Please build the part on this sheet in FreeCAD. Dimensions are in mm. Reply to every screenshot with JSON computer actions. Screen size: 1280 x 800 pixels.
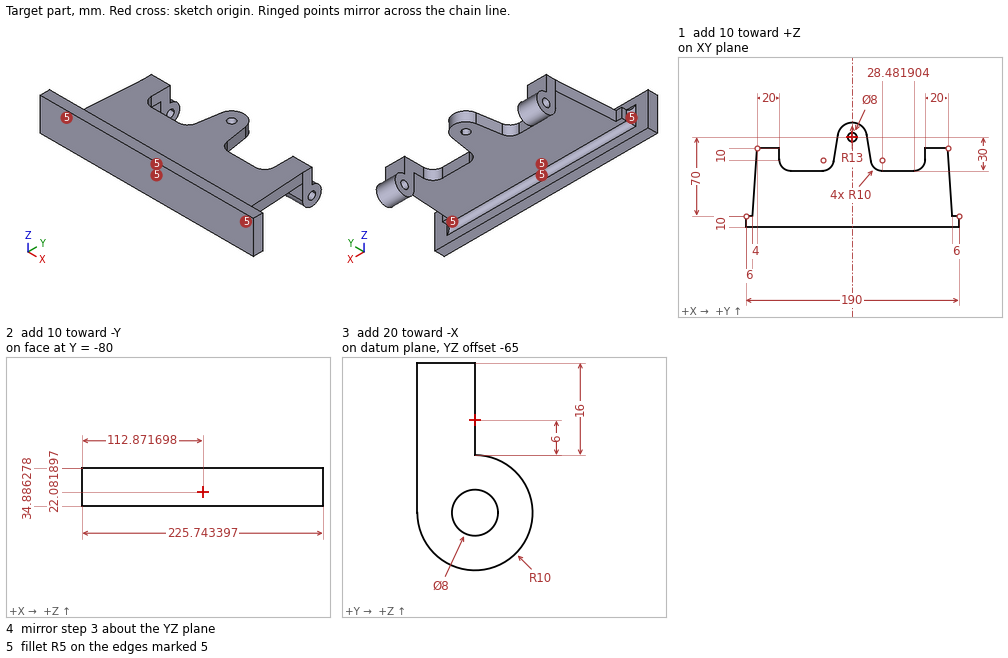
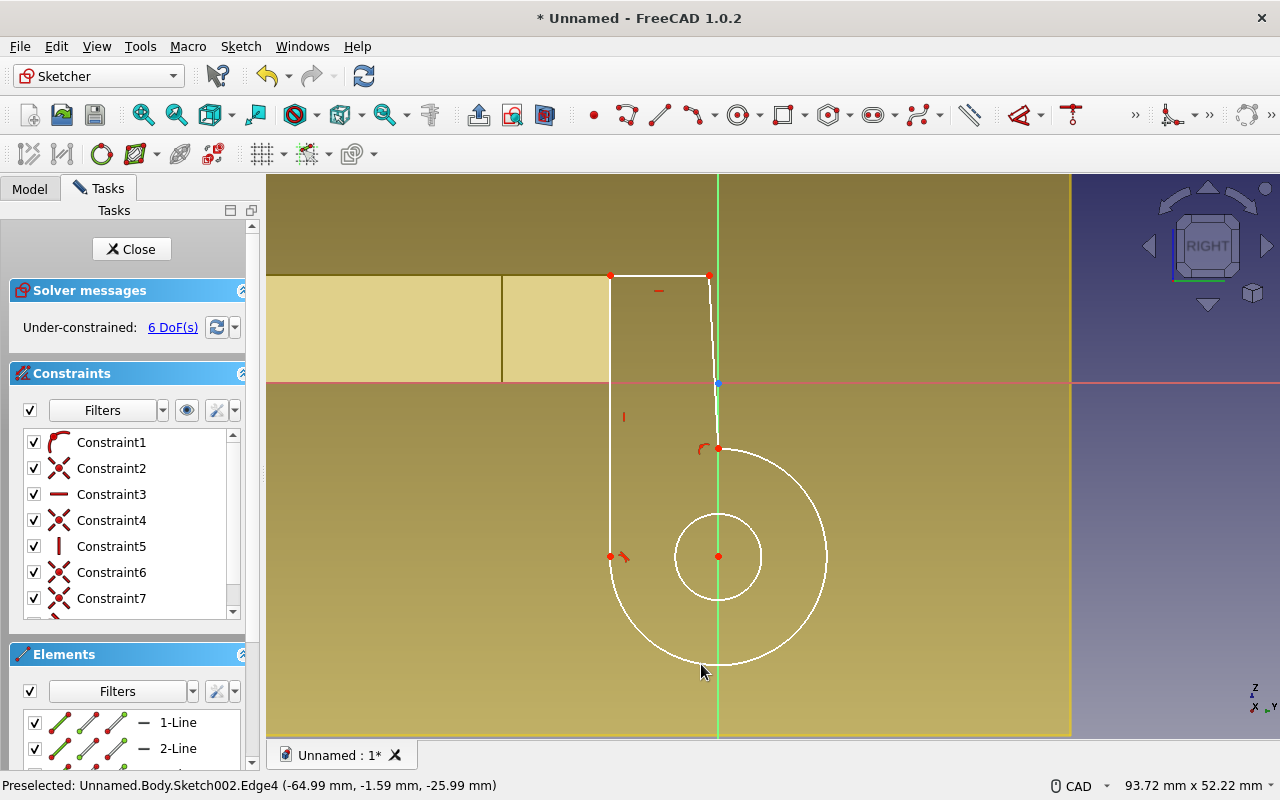
{"action": "left_click", "coordinate": [716, 397]}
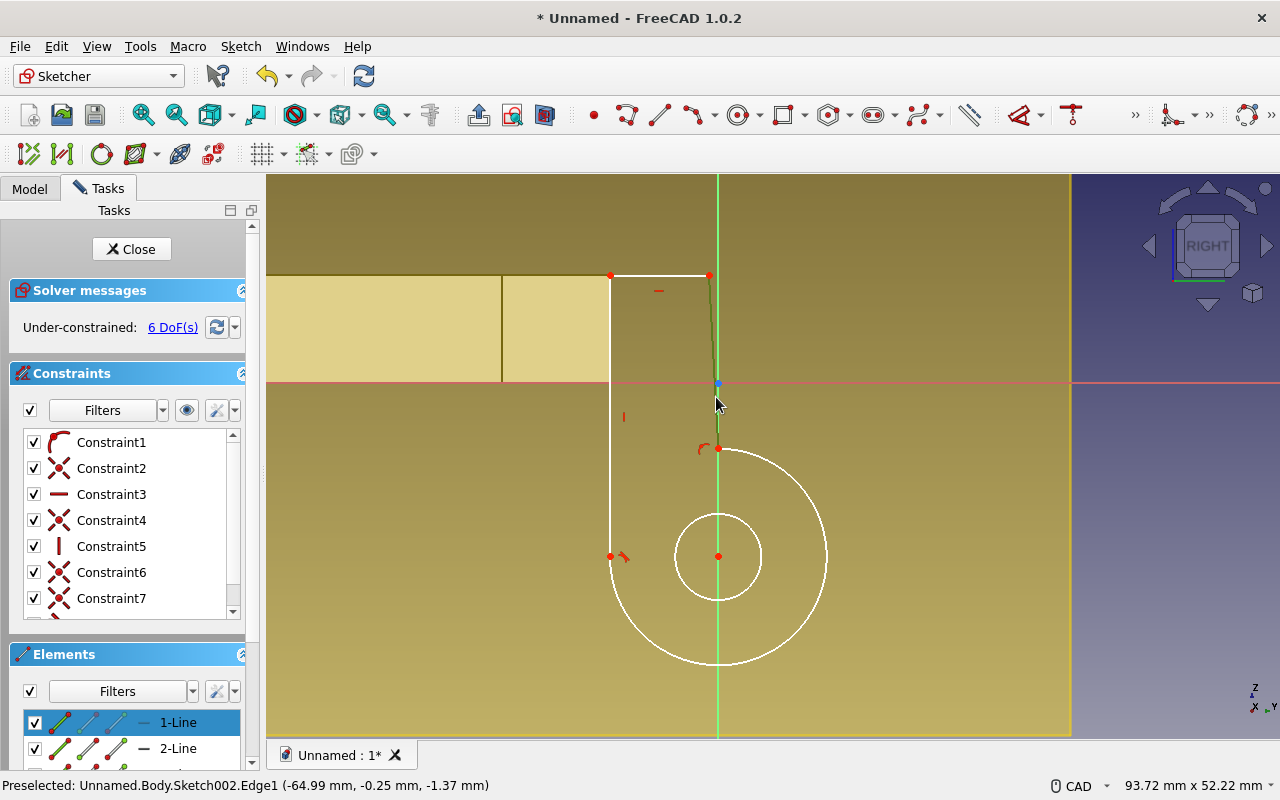
{"action": "key", "text": "v"}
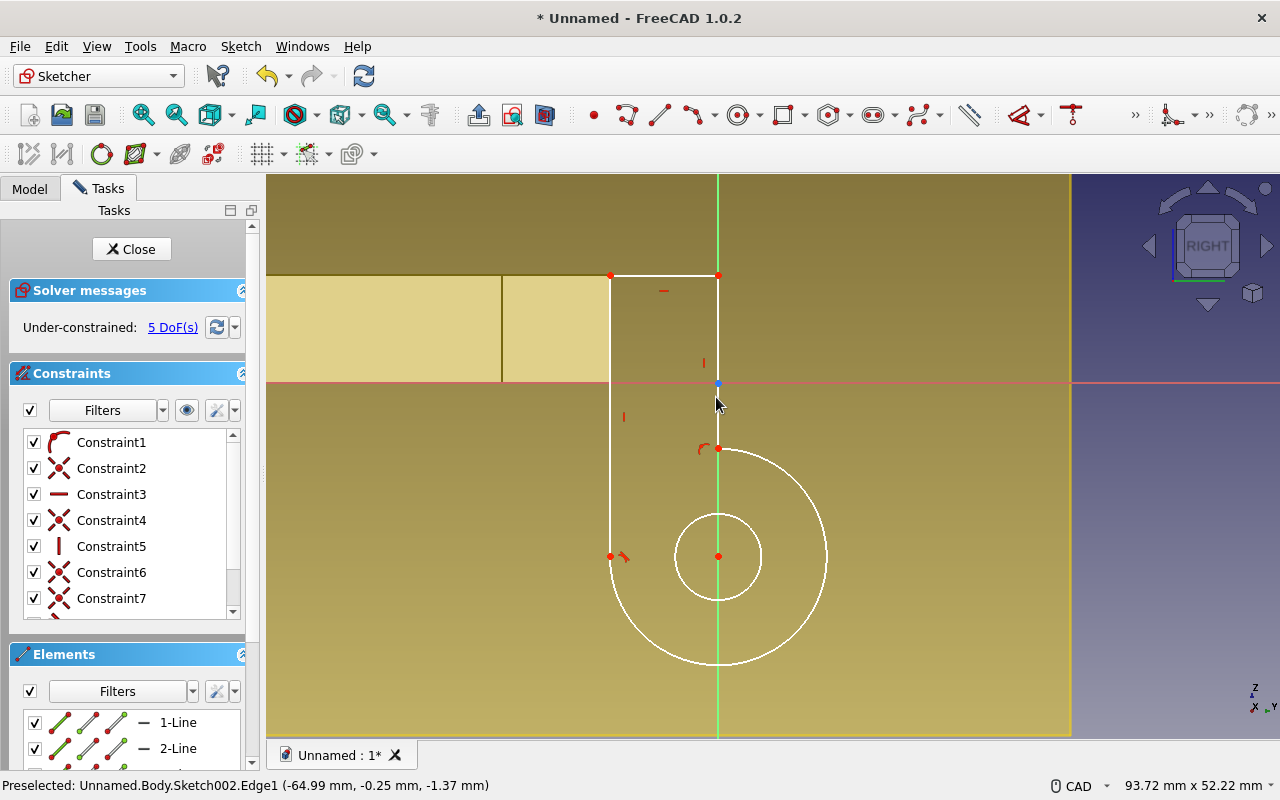
{"action": "left_click", "coordinate": [718, 557]}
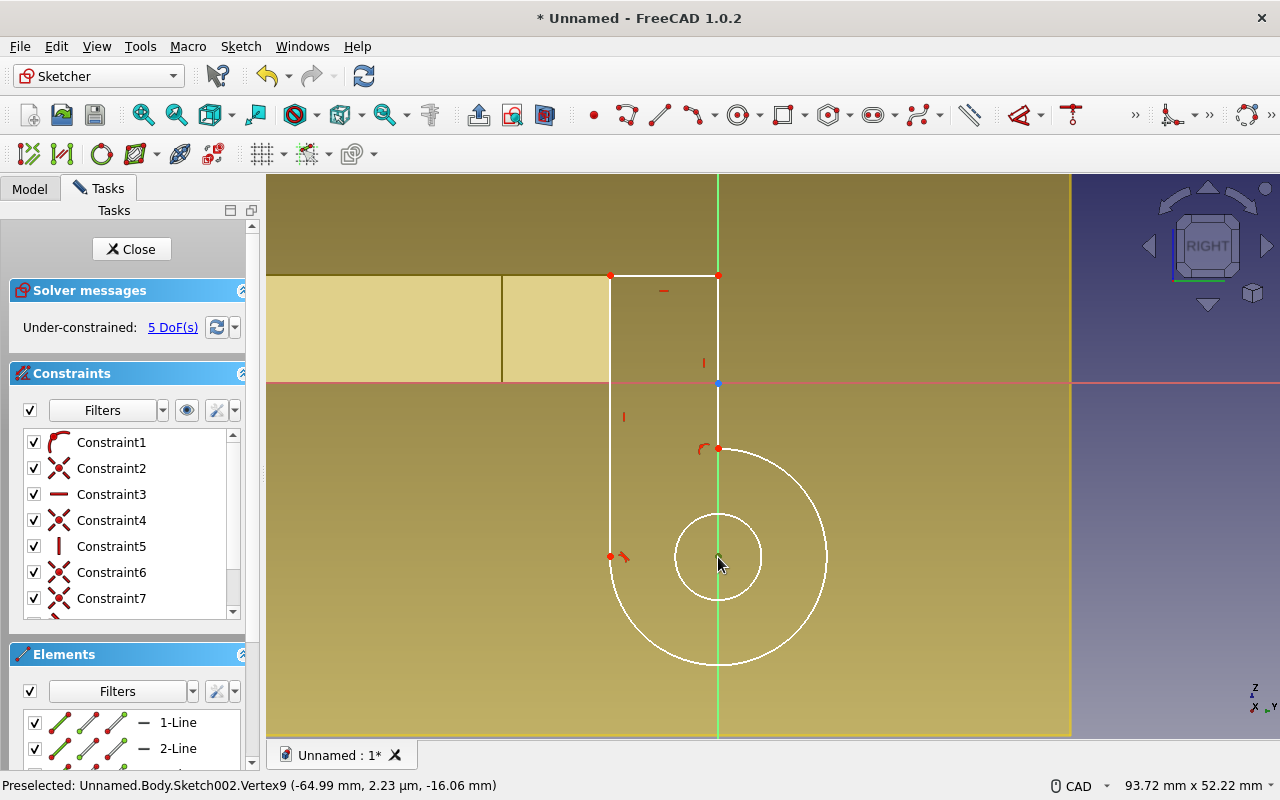
{"action": "left_click", "coordinate": [718, 566]}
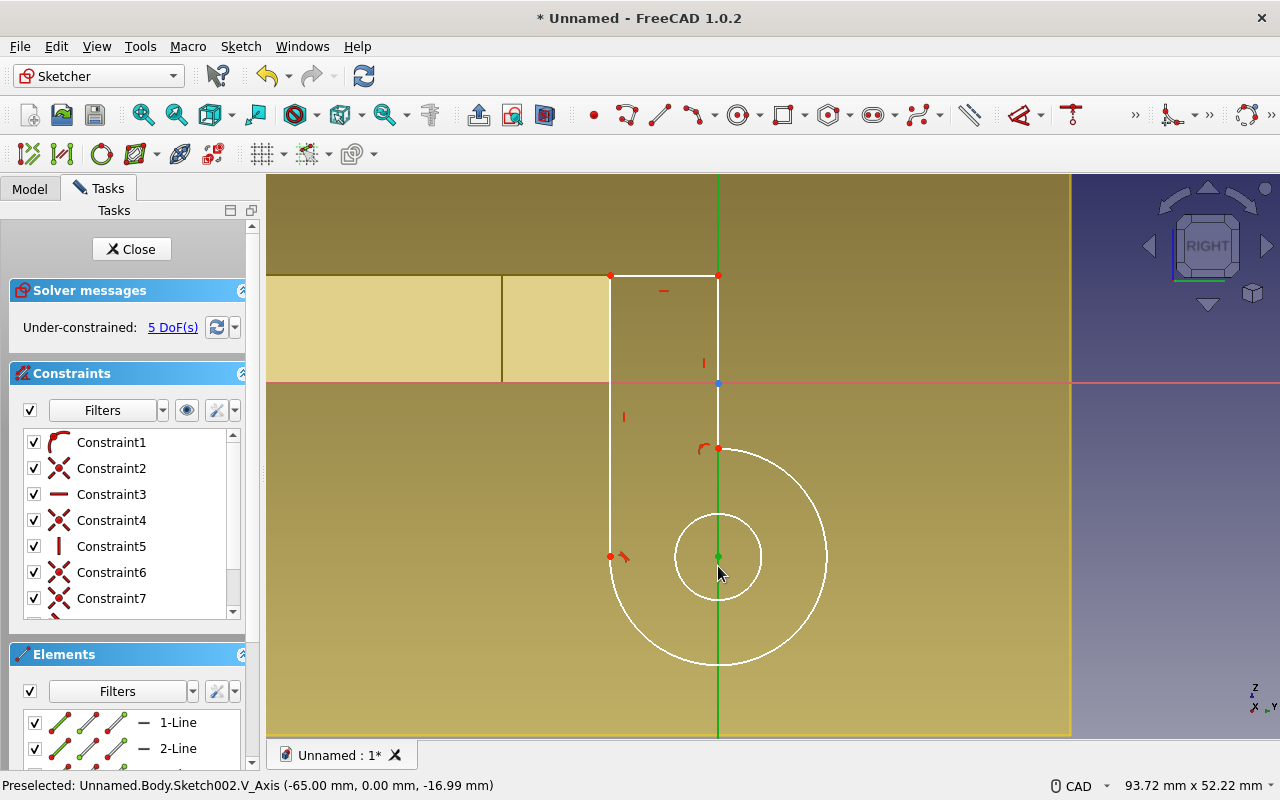
{"action": "left_click", "coordinate": [1071, 116]}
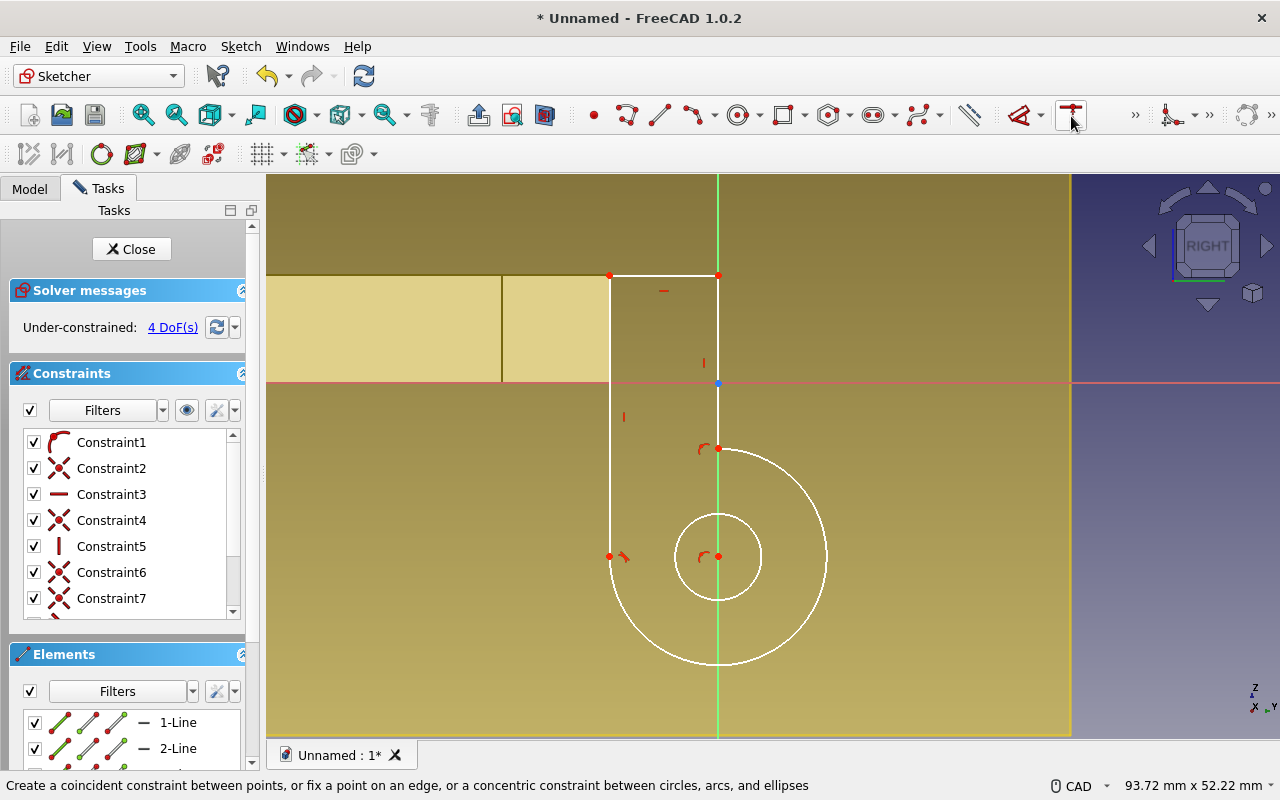
{"action": "key", "text": "d"}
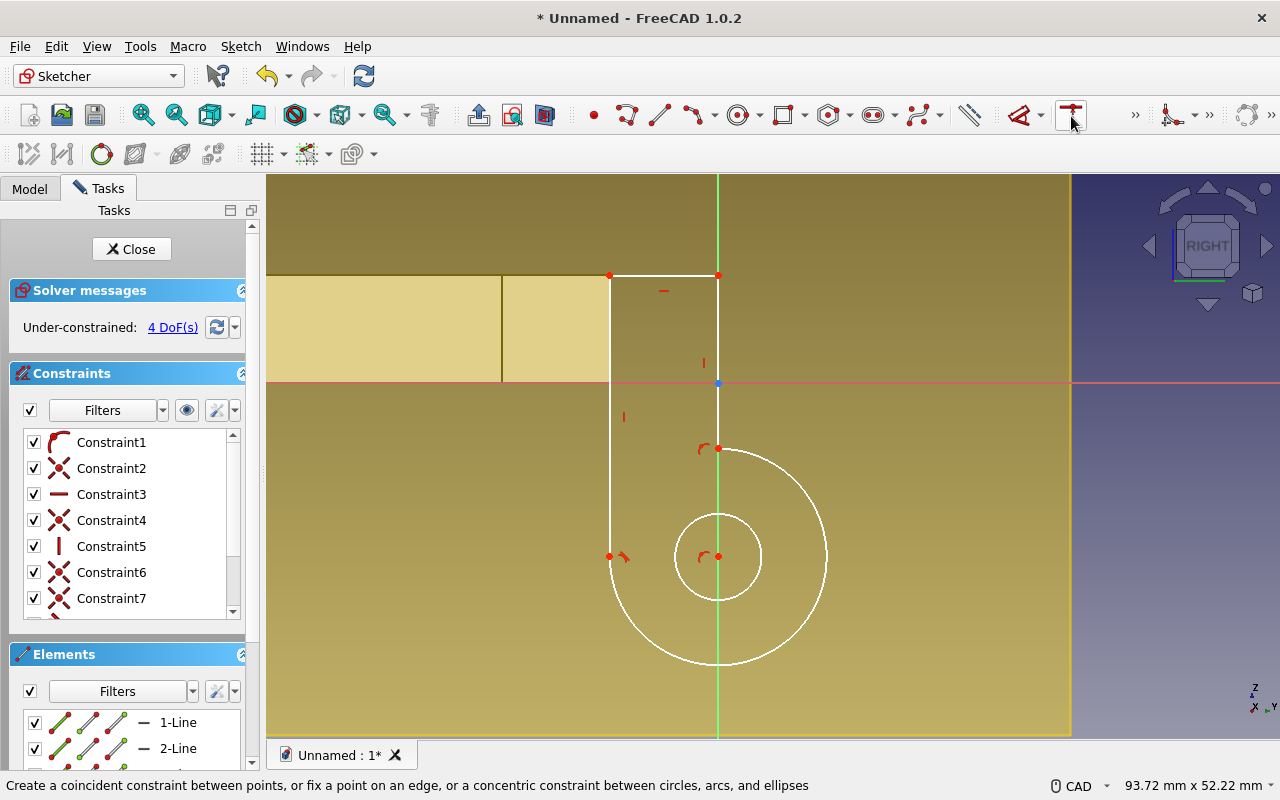
{"action": "left_click", "coordinate": [701, 664]}
{"action": "left_click", "coordinate": [696, 696]}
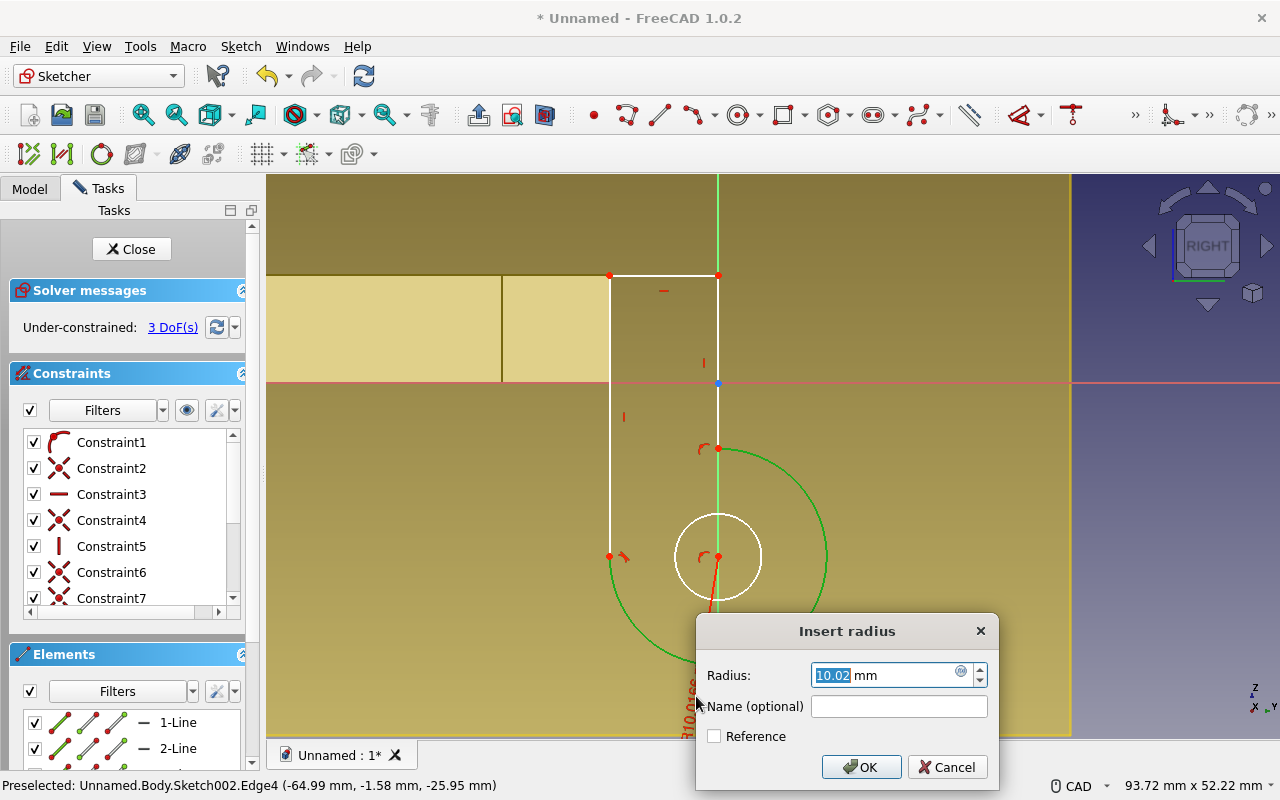
{"action": "type", "text": "10"}
{"action": "key", "text": "Return"}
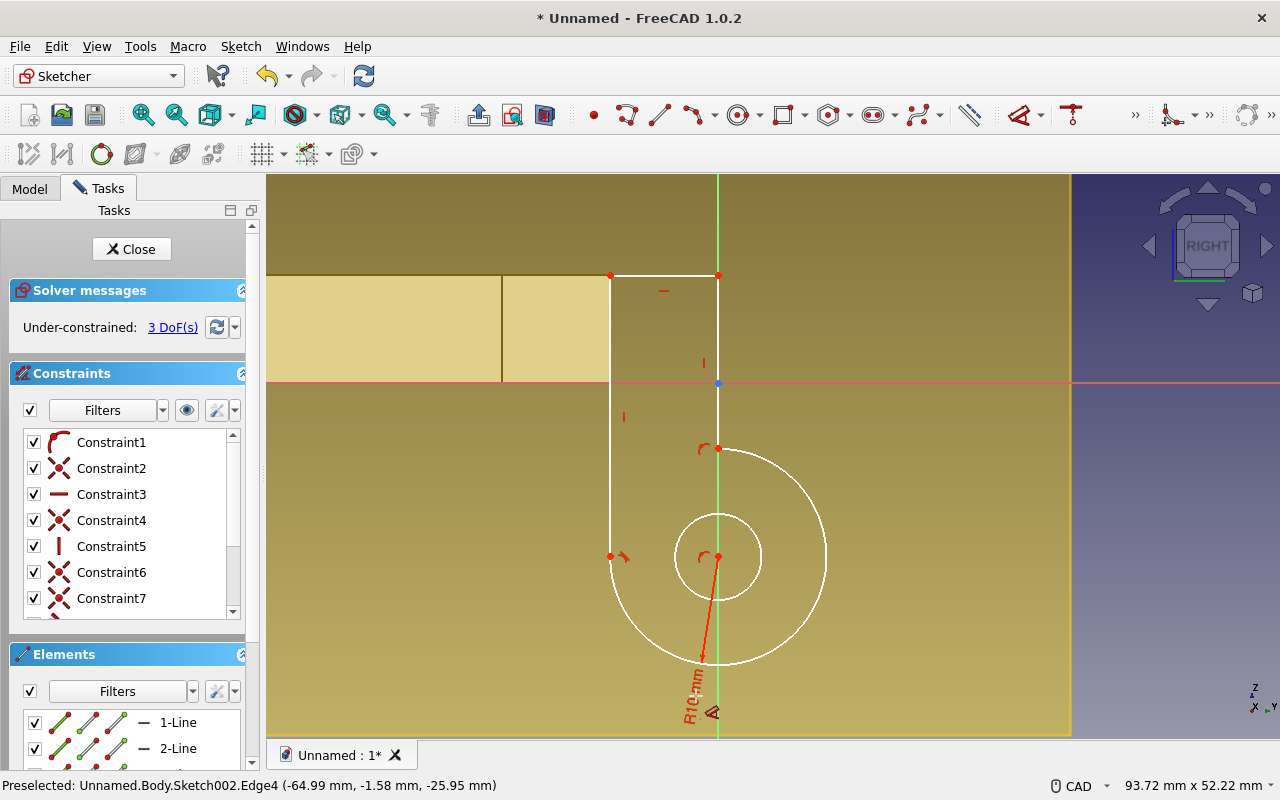
{"action": "left_click", "coordinate": [749, 526]}
{"action": "left_click", "coordinate": [772, 503]}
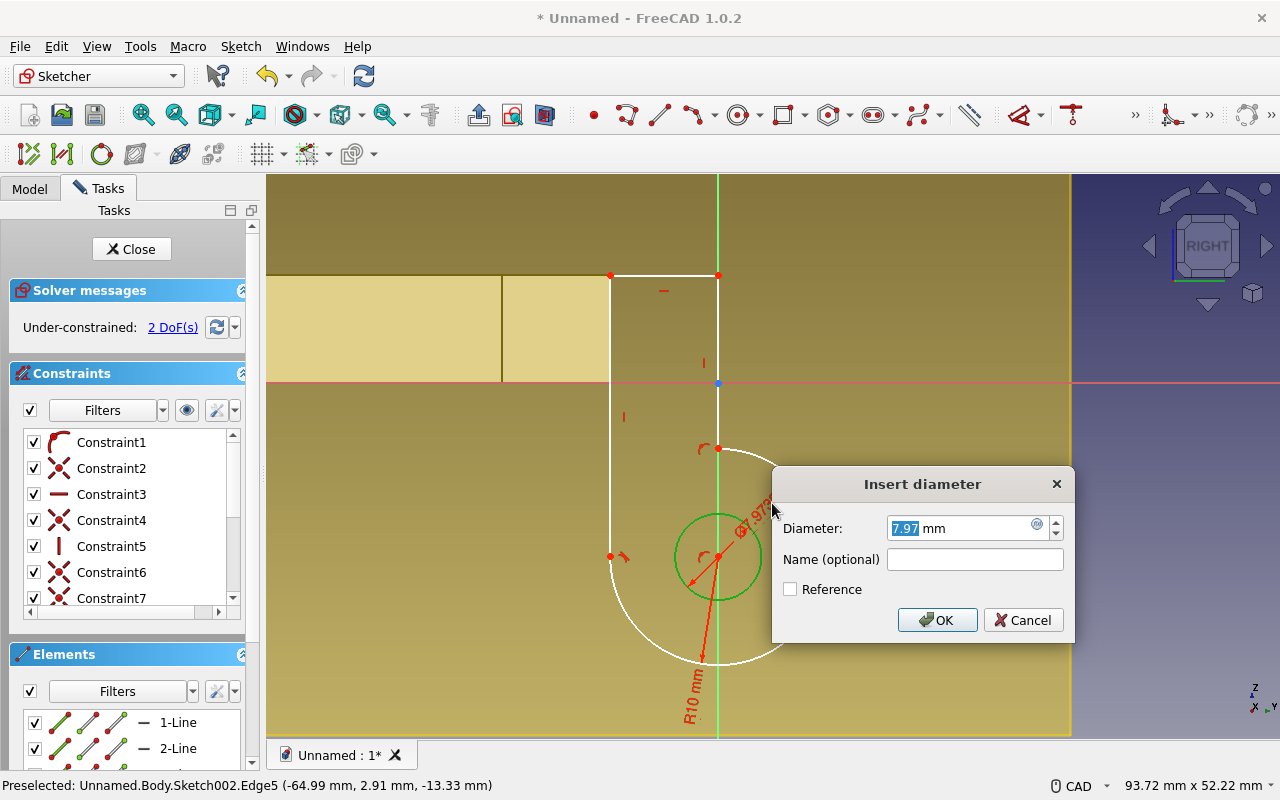
{"action": "type", "text": "8"}
{"action": "key", "text": "Return"}